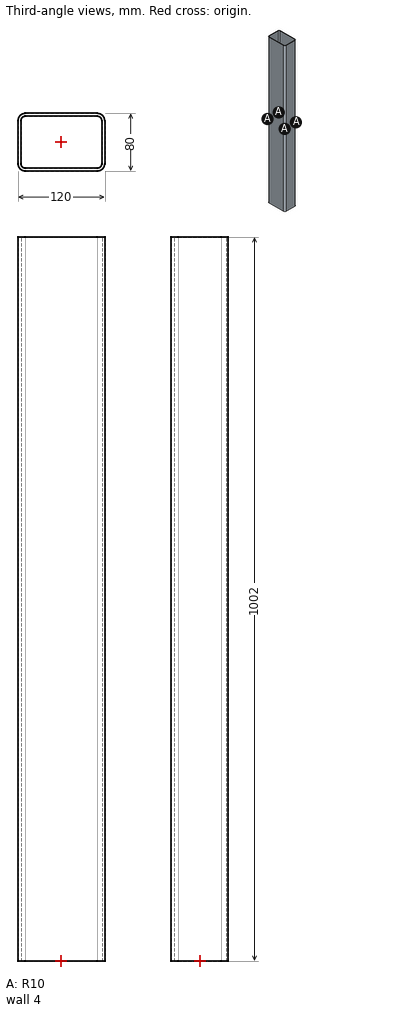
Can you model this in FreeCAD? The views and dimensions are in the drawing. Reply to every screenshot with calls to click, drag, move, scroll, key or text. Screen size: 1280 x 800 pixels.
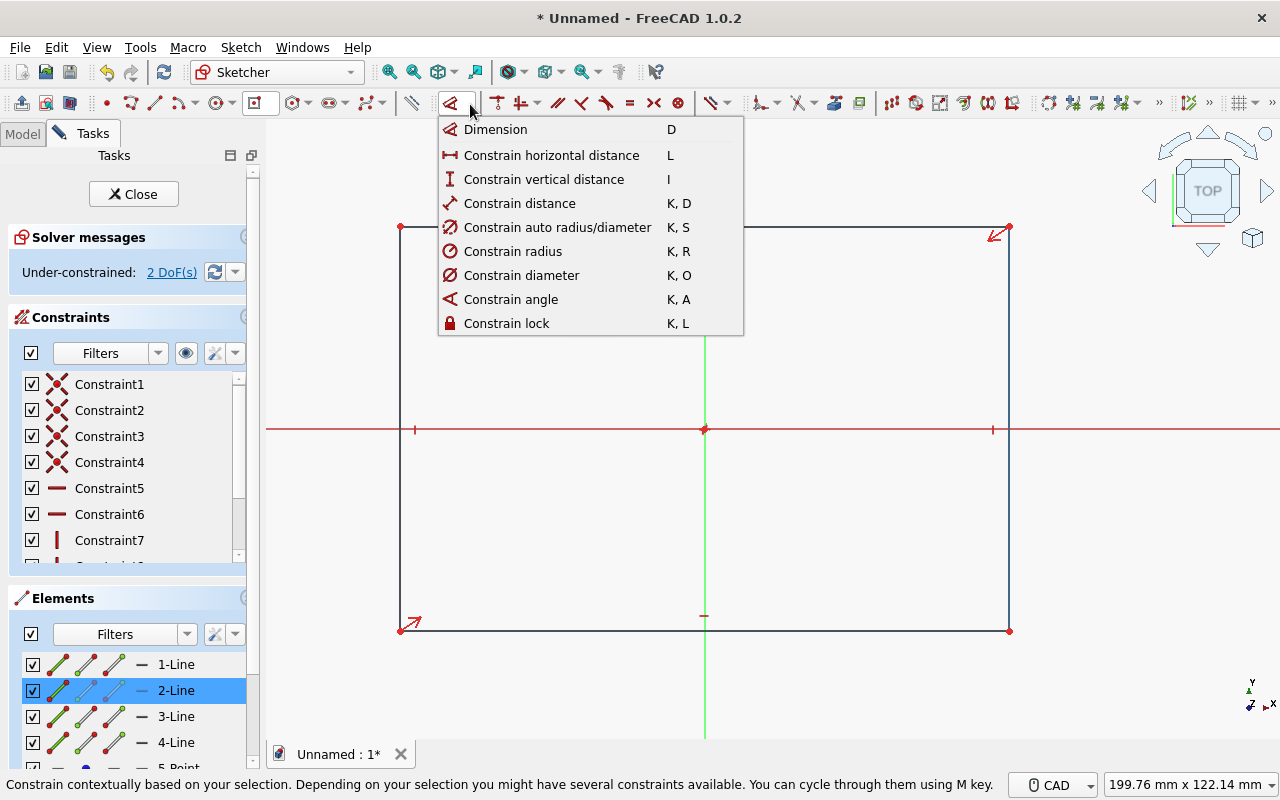
click(591, 179)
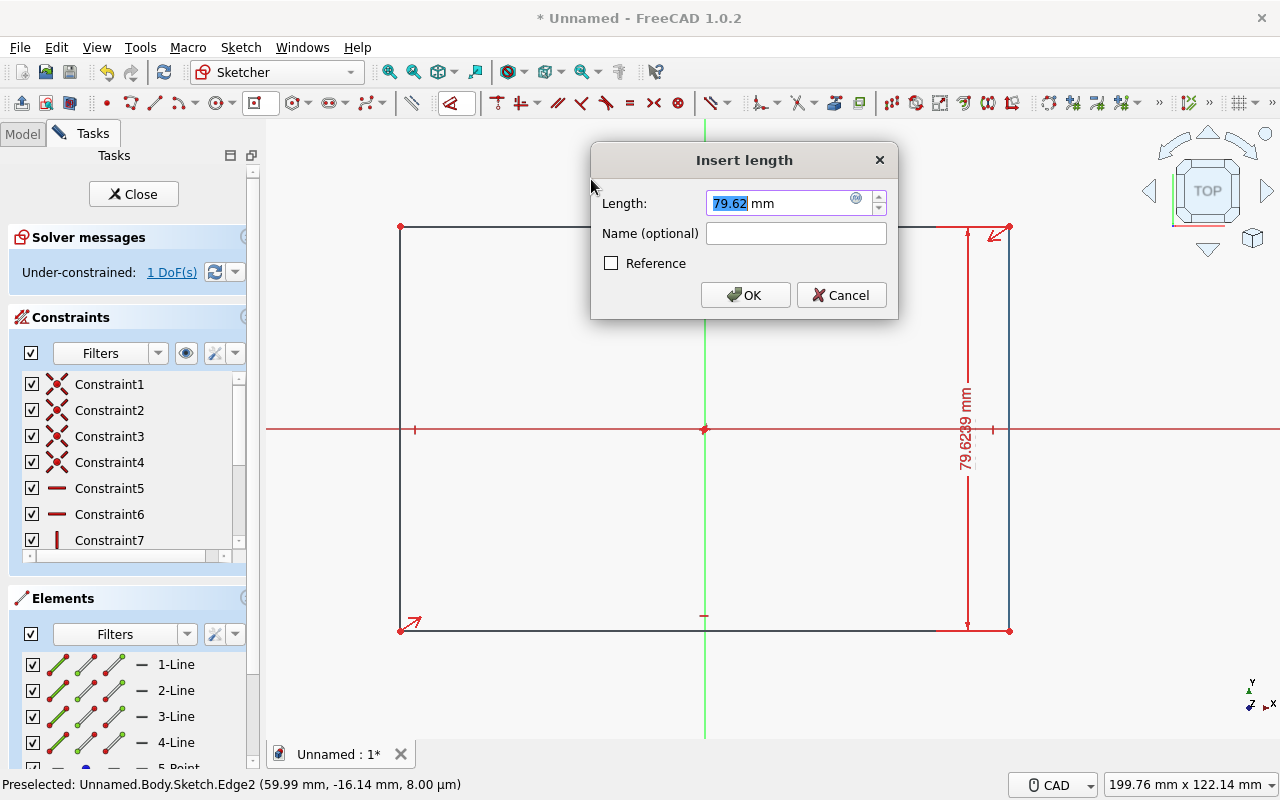
text(80)
key(Return)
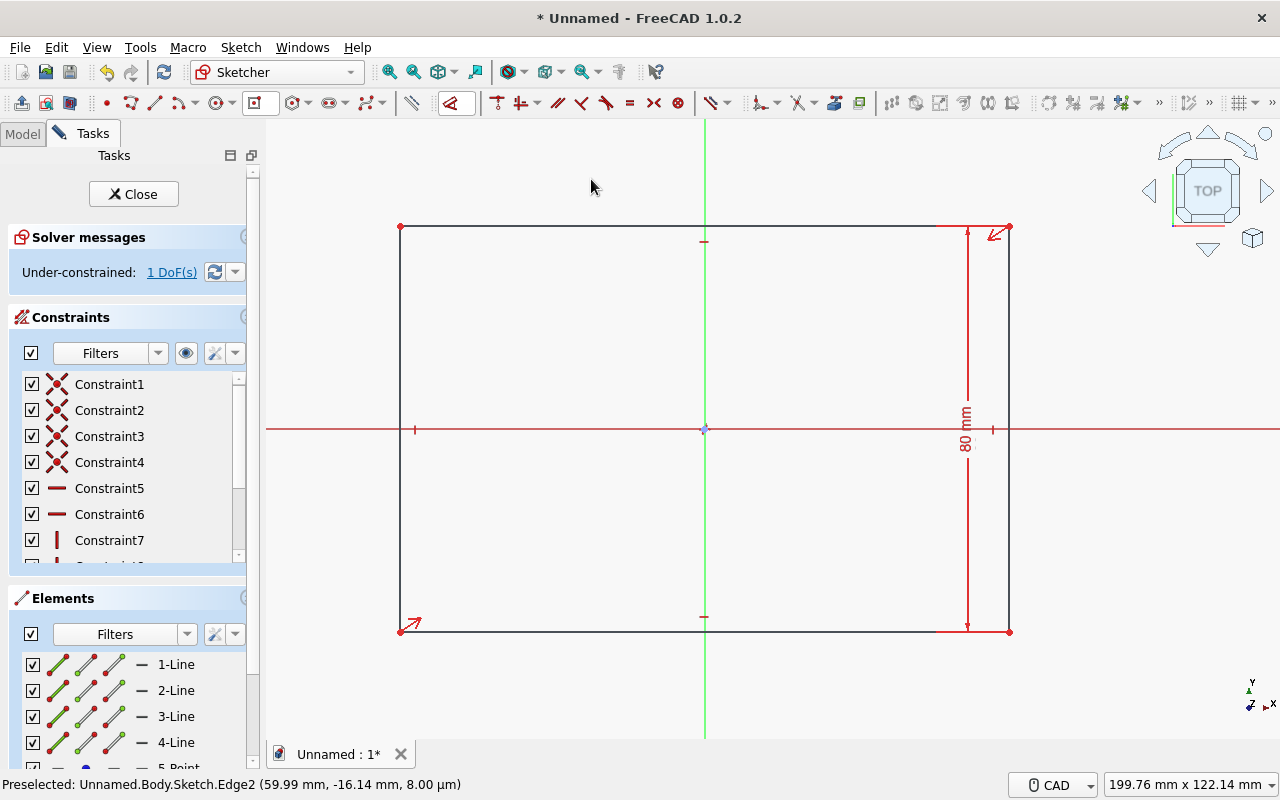
click(583, 632)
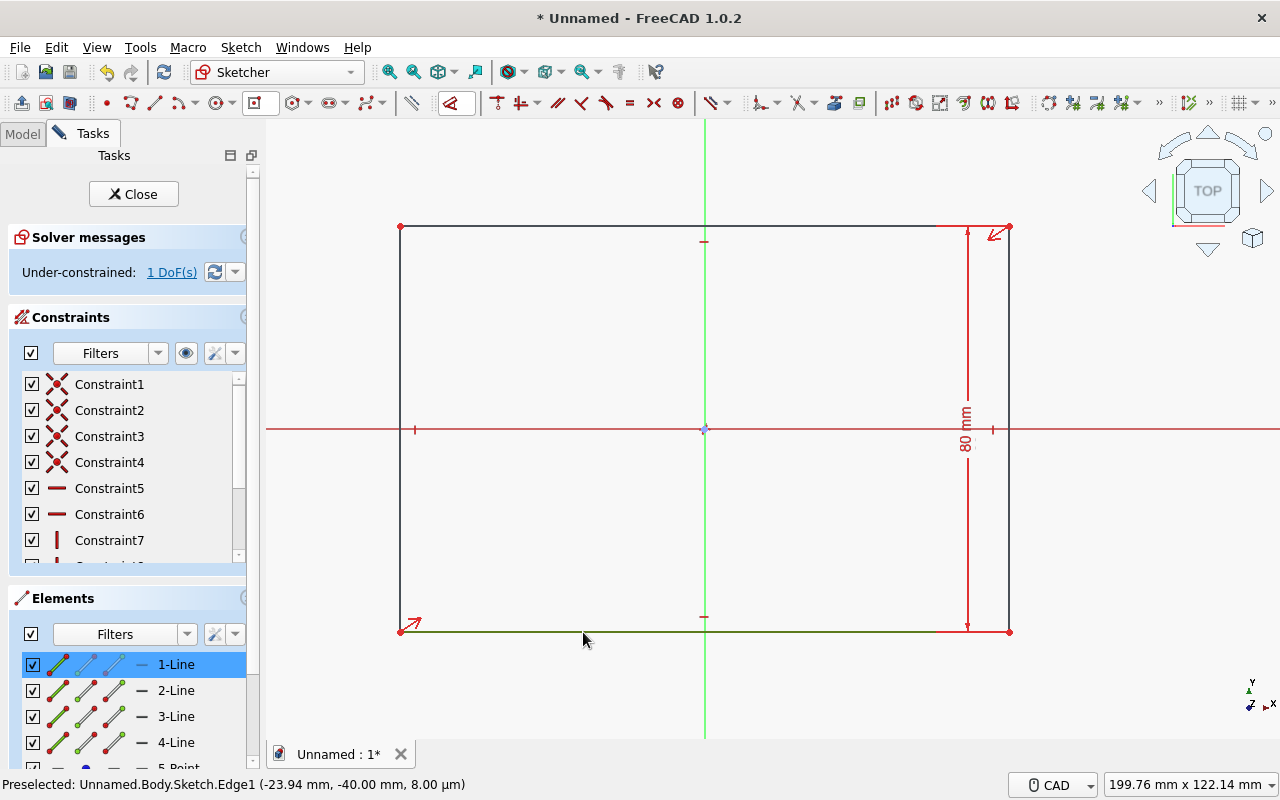
click(470, 104)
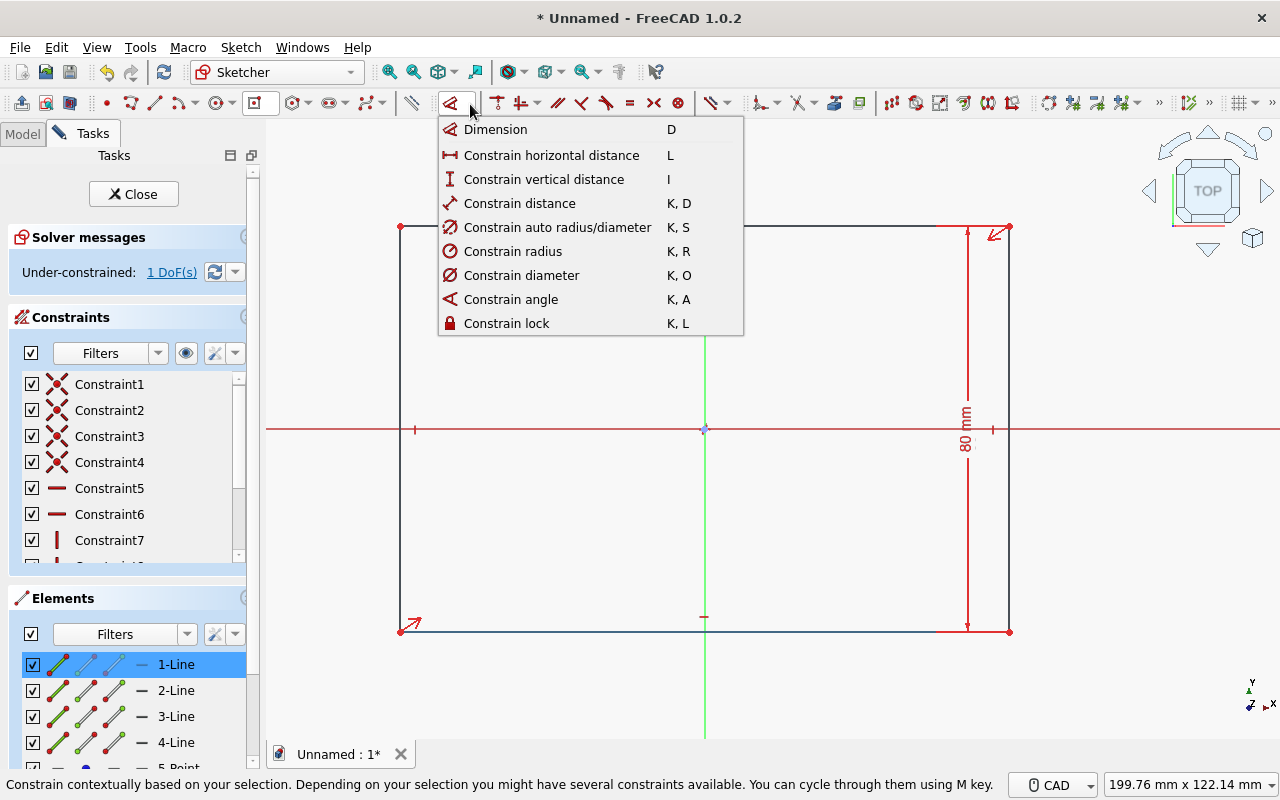
click(591, 155)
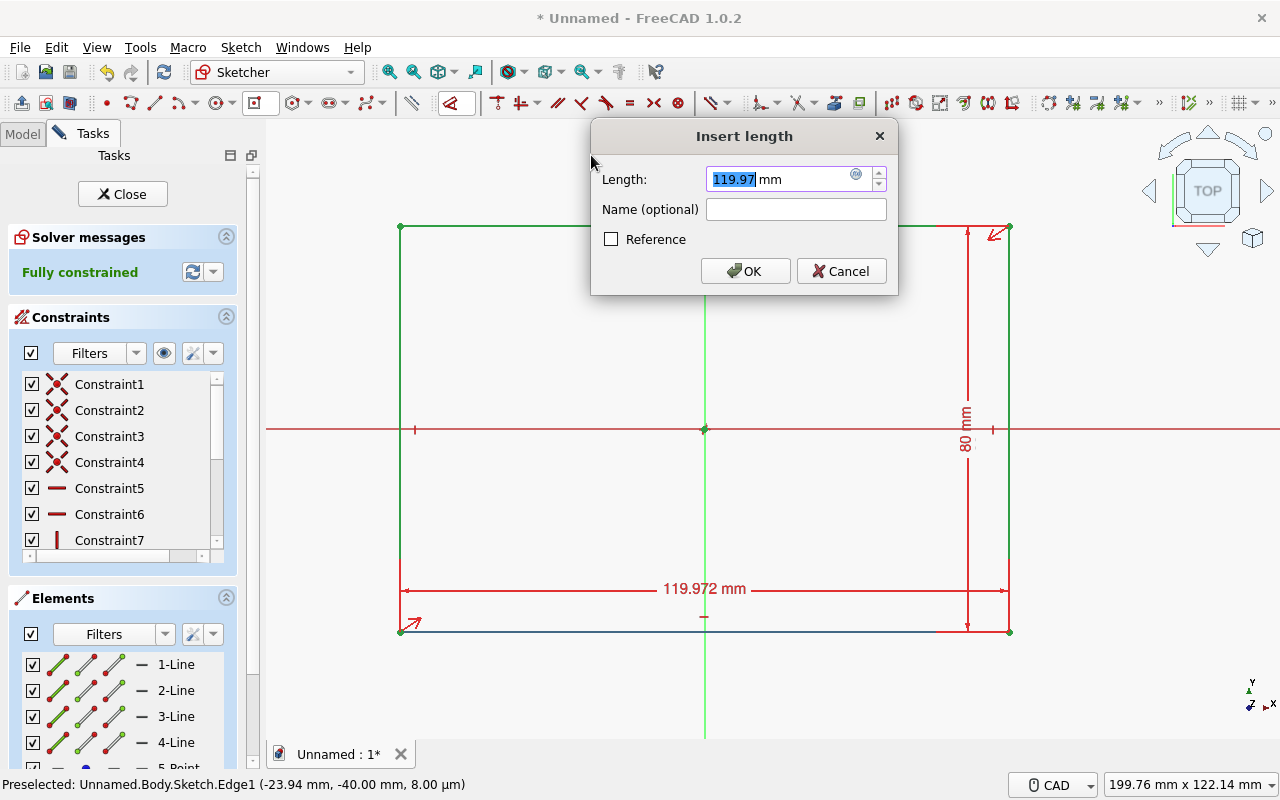
text(120)
key(Return)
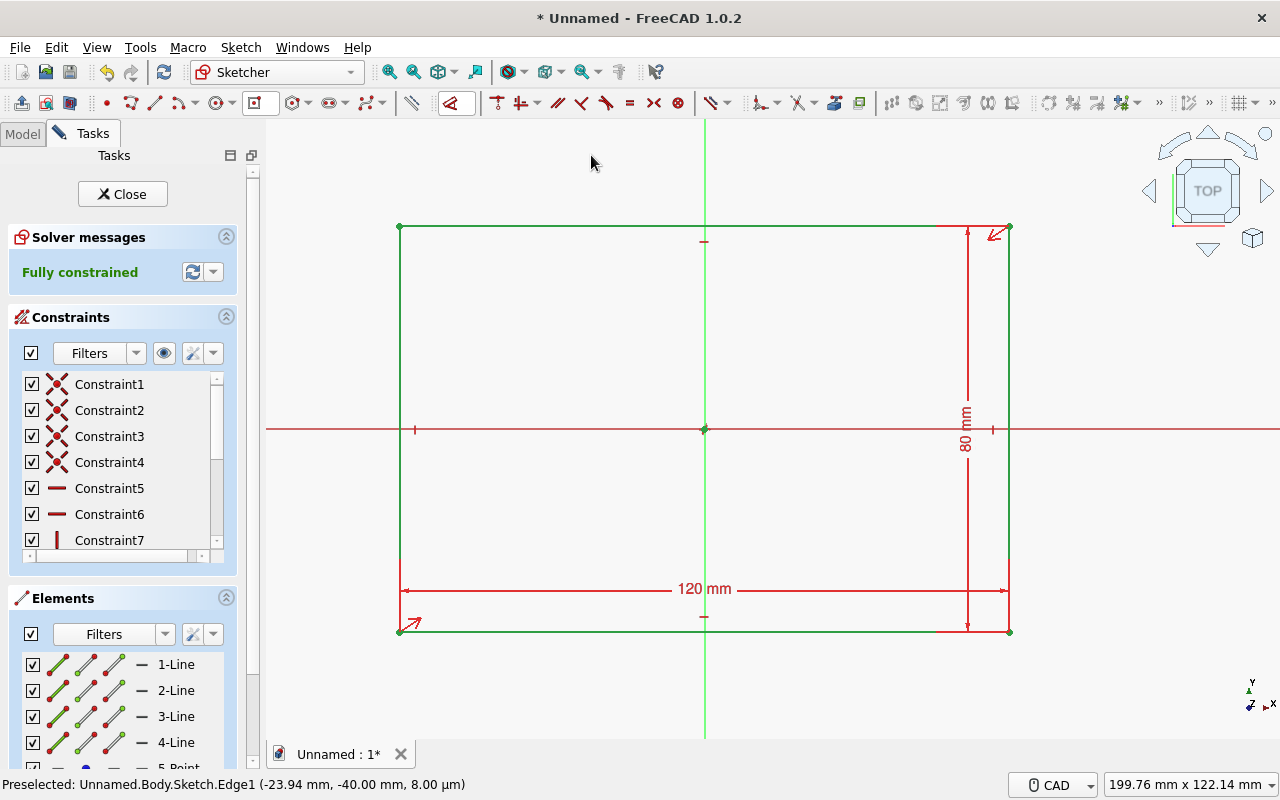
click(123, 194)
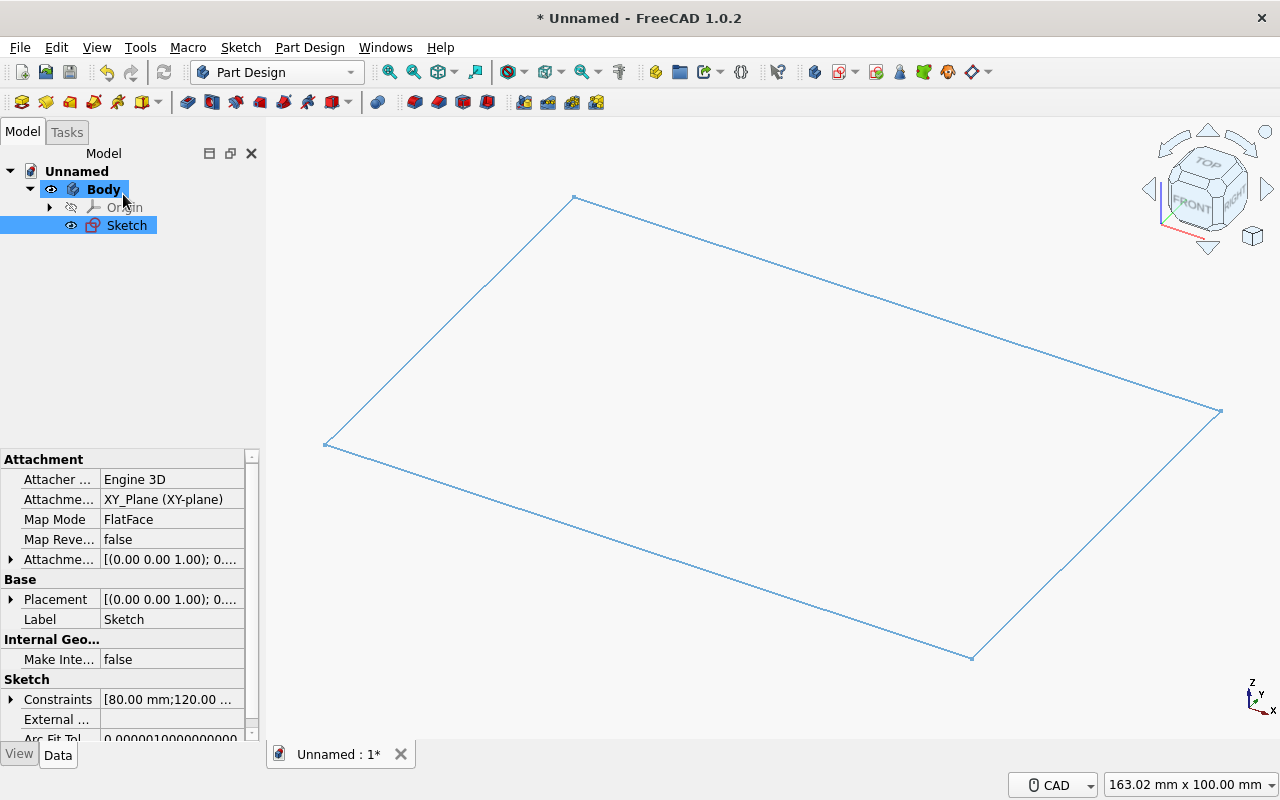
click(22, 102)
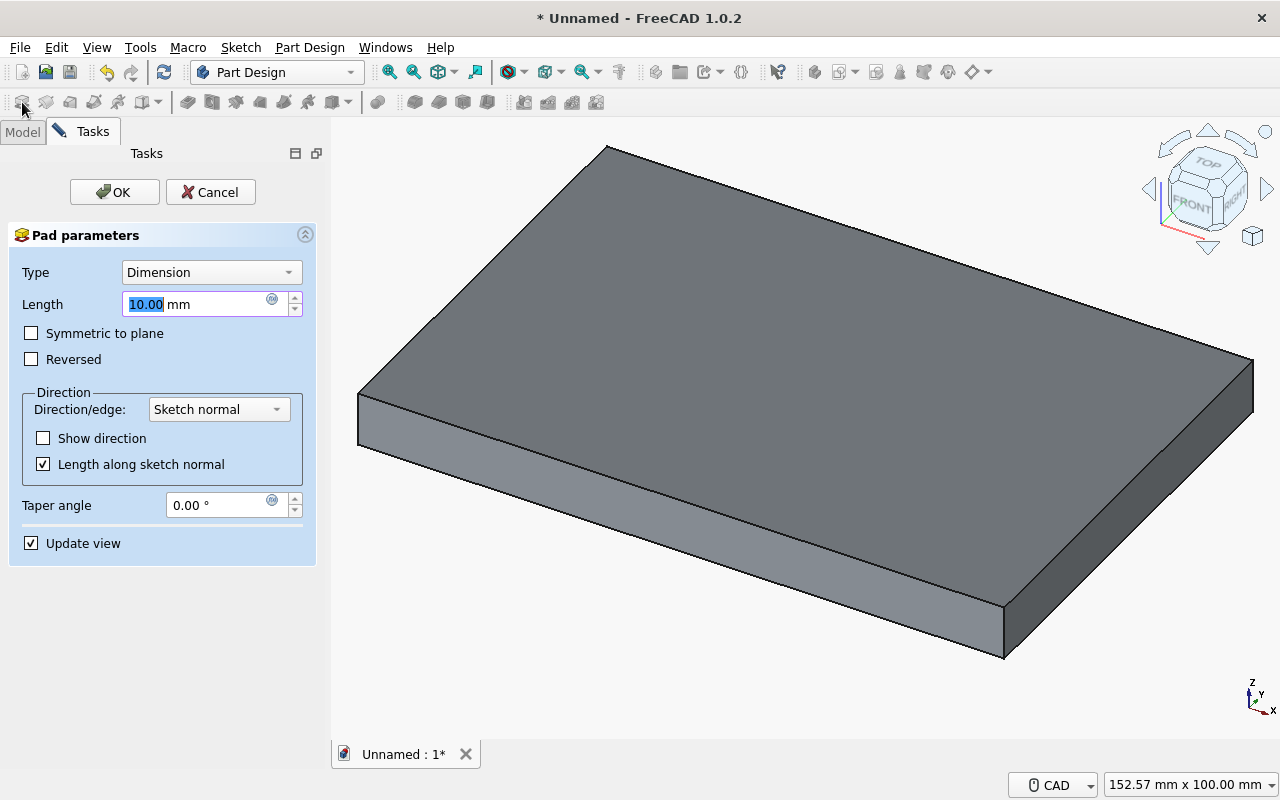
text(1002)
key(Tab)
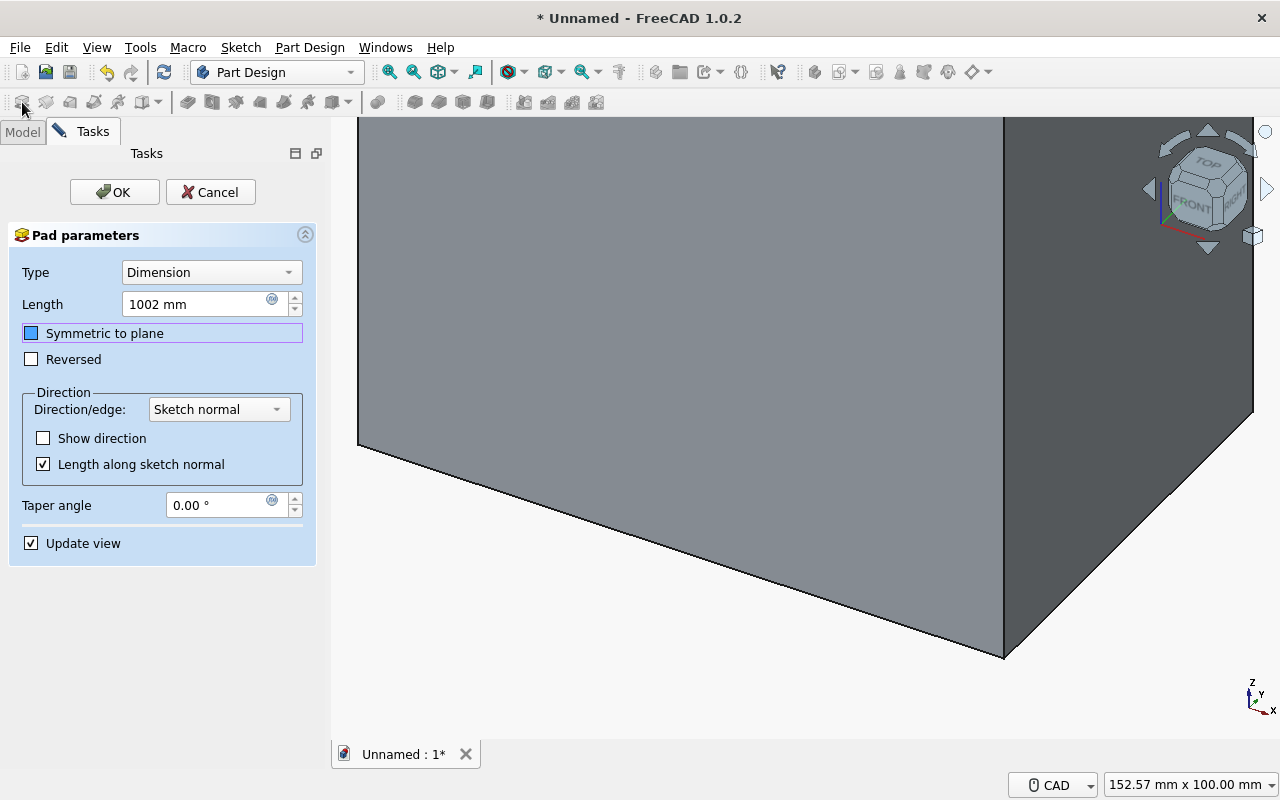
click(115, 192)